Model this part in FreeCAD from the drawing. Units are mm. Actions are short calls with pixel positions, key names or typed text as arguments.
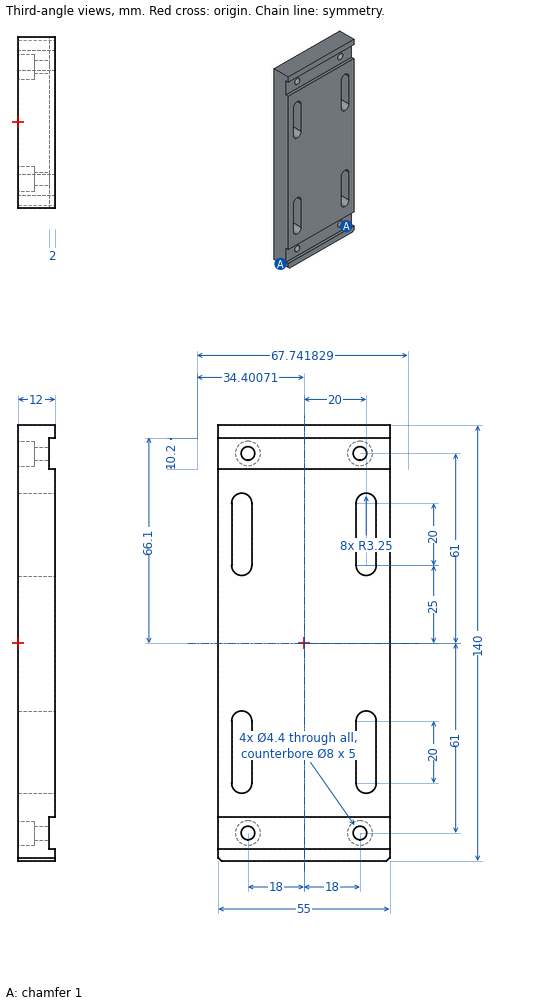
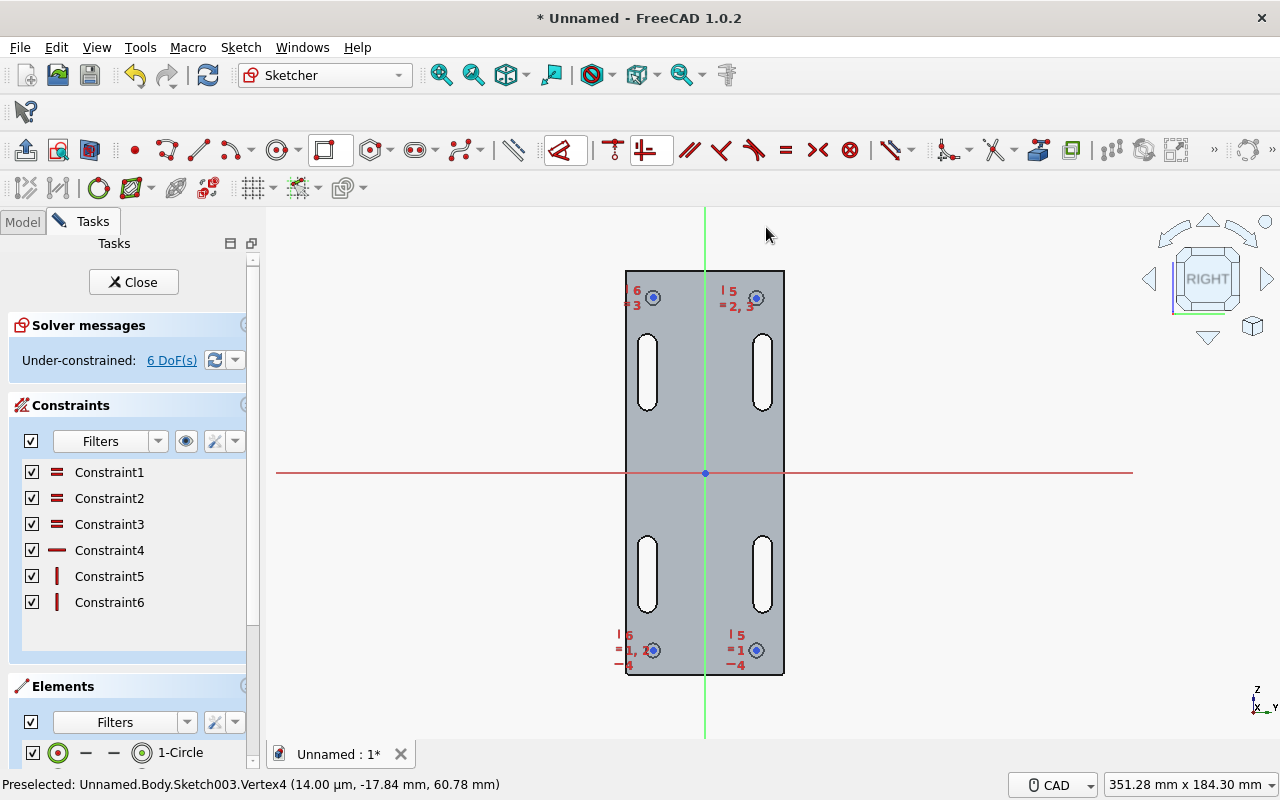
click(757, 298)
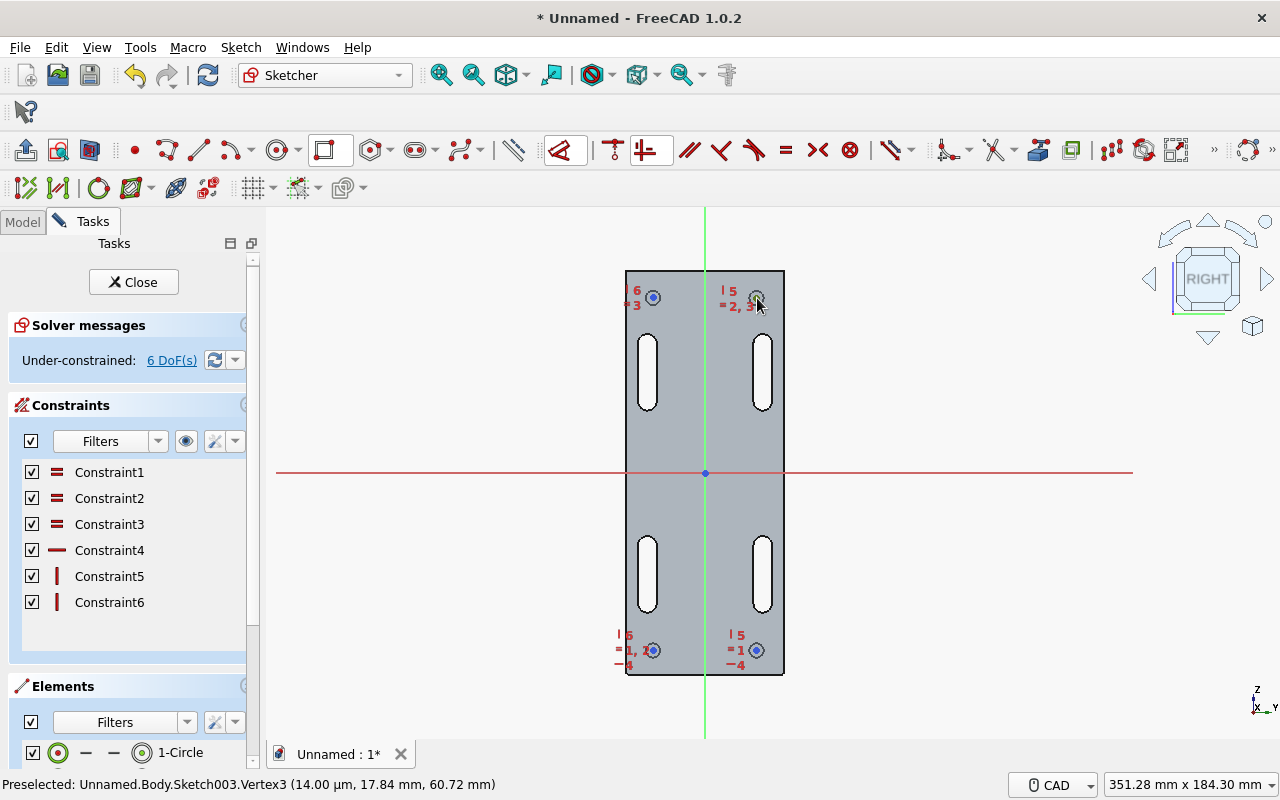
click(653, 298)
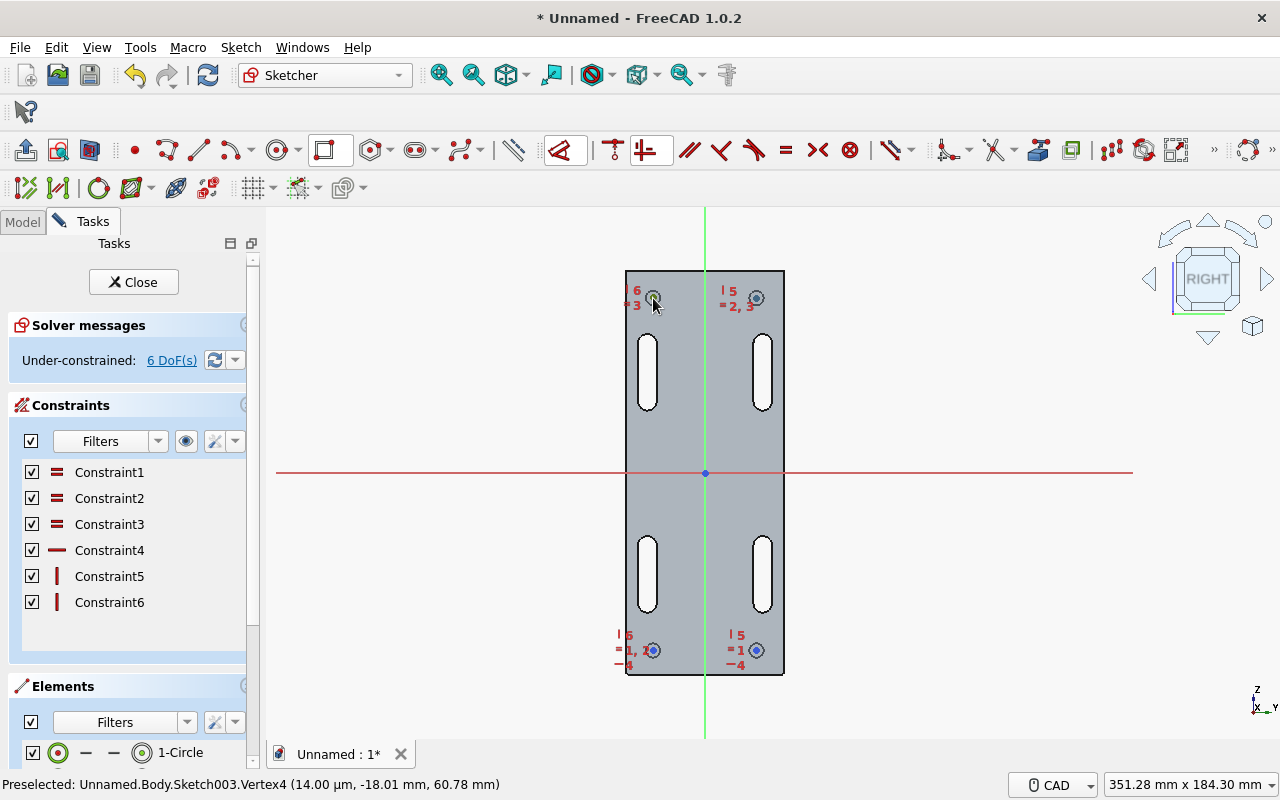
click(668, 150)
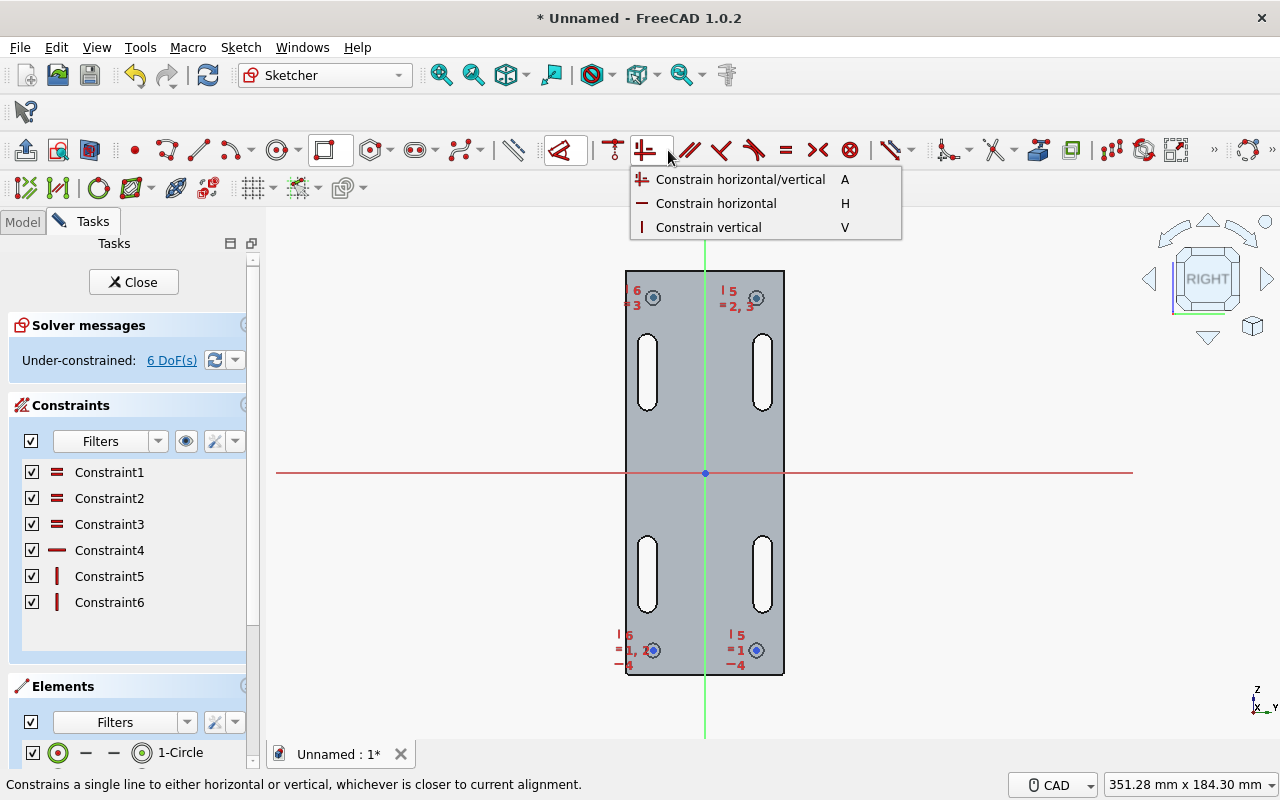
click(766, 203)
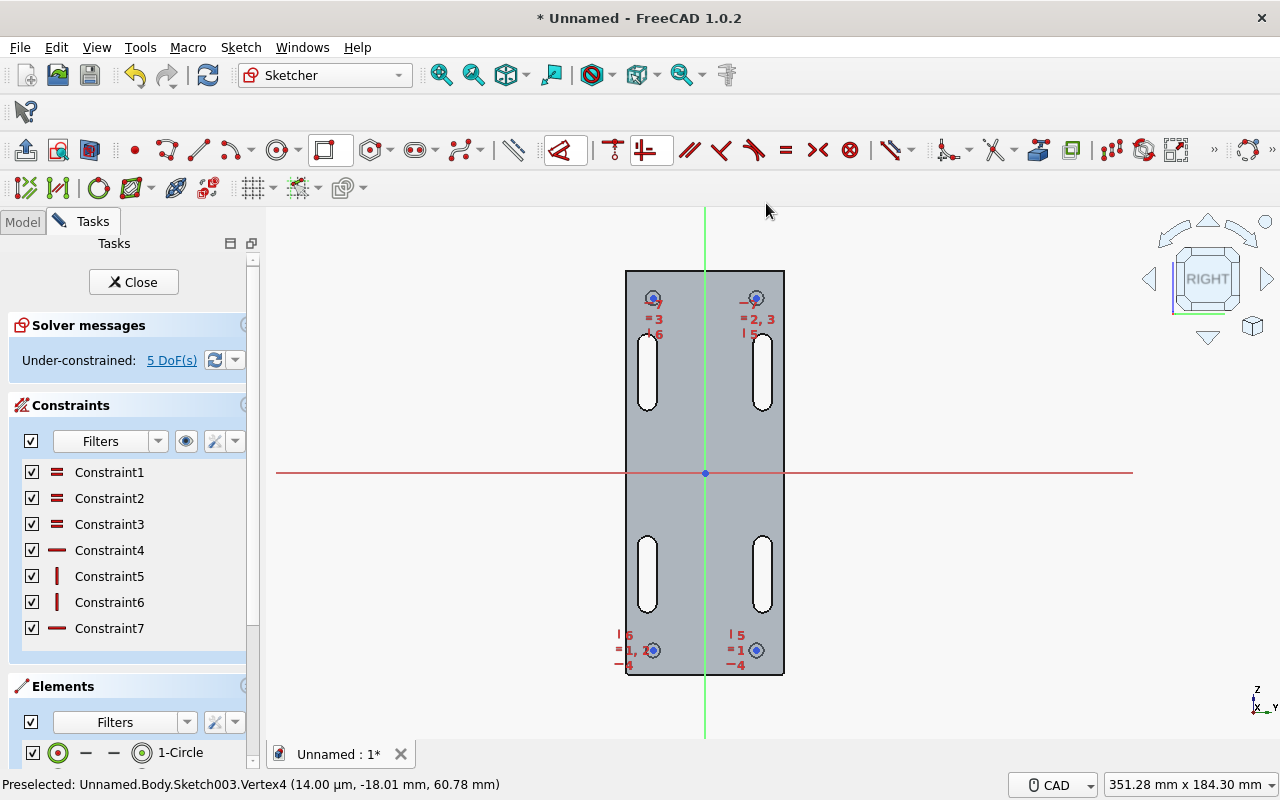
scroll(751, 645, up, 6)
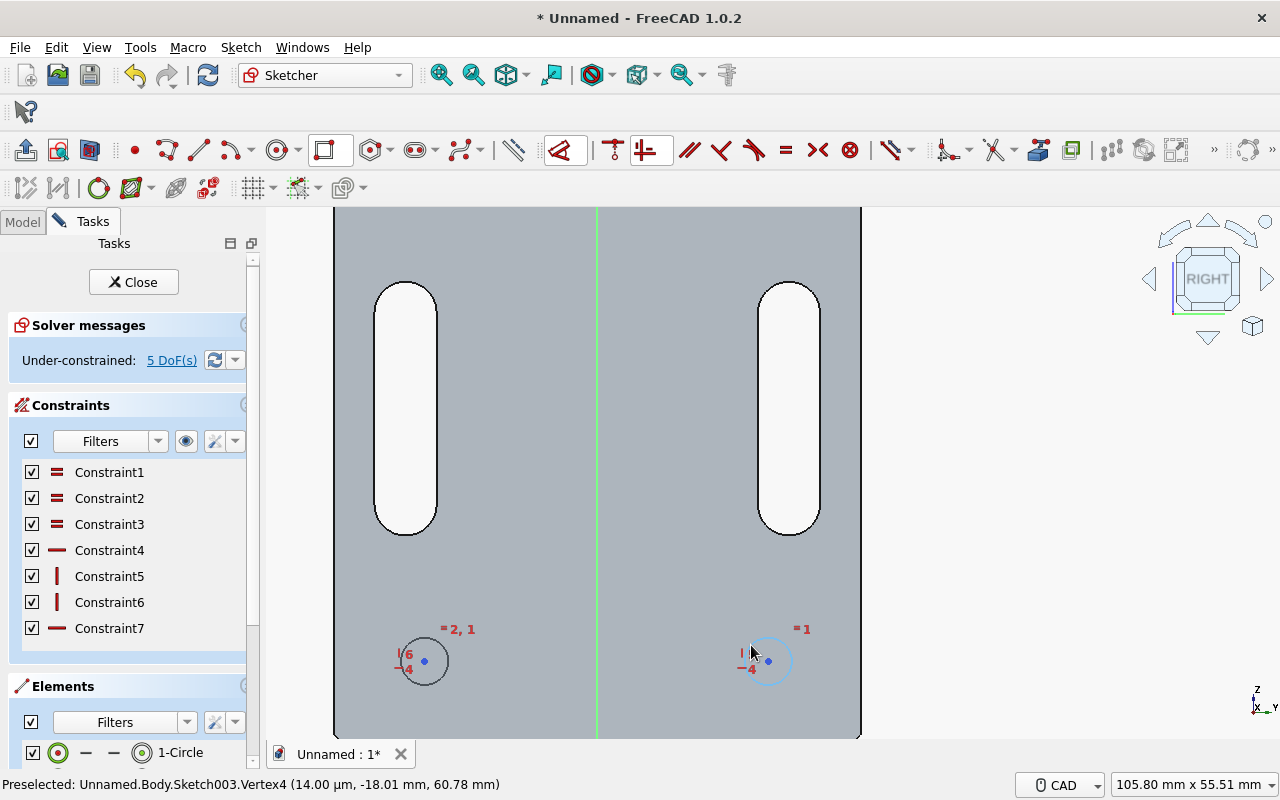
click(752, 645)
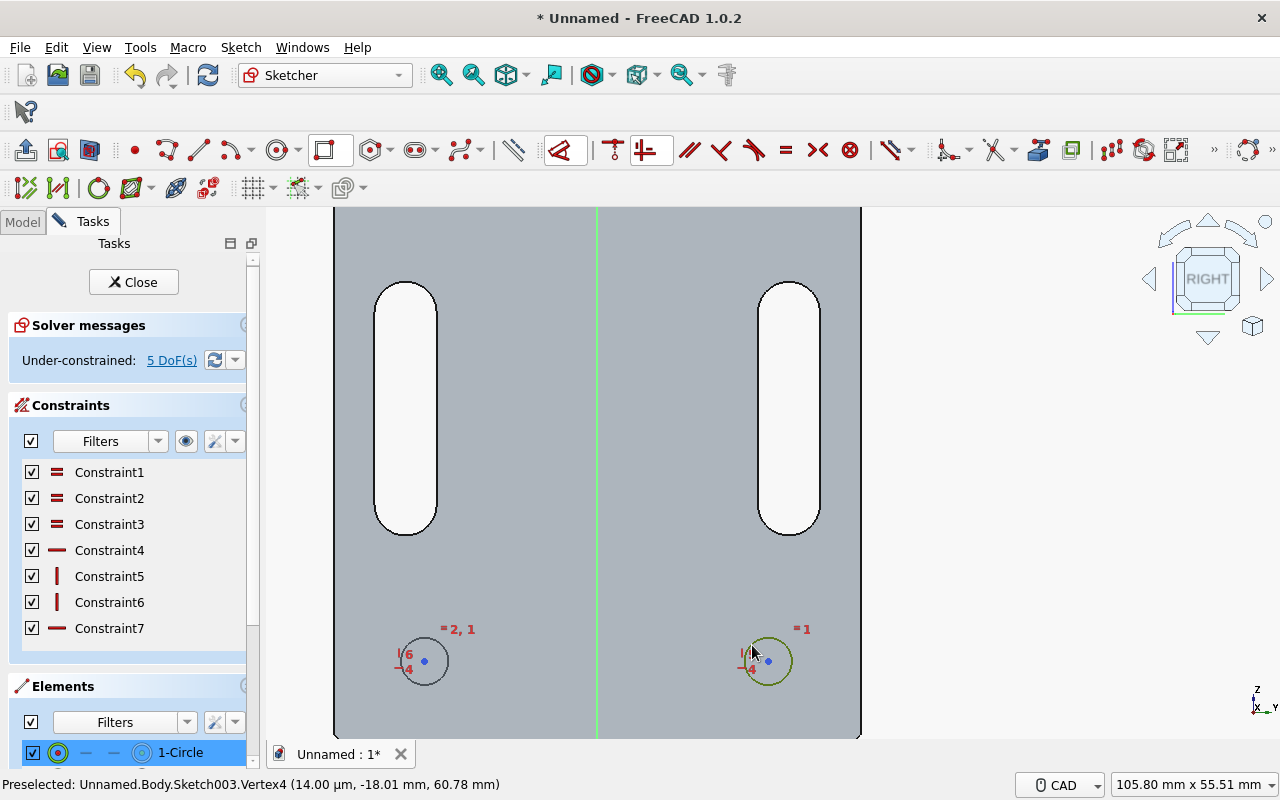
click(582, 150)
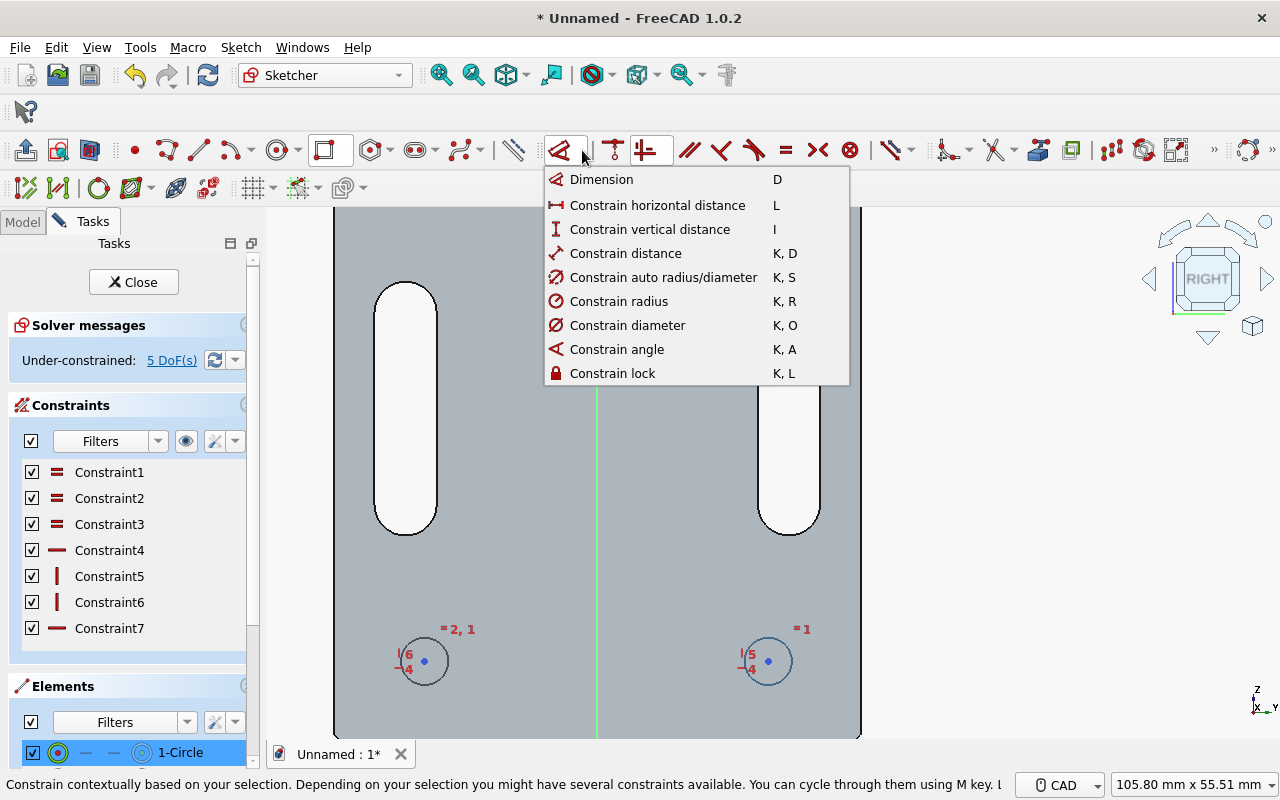
click(697, 325)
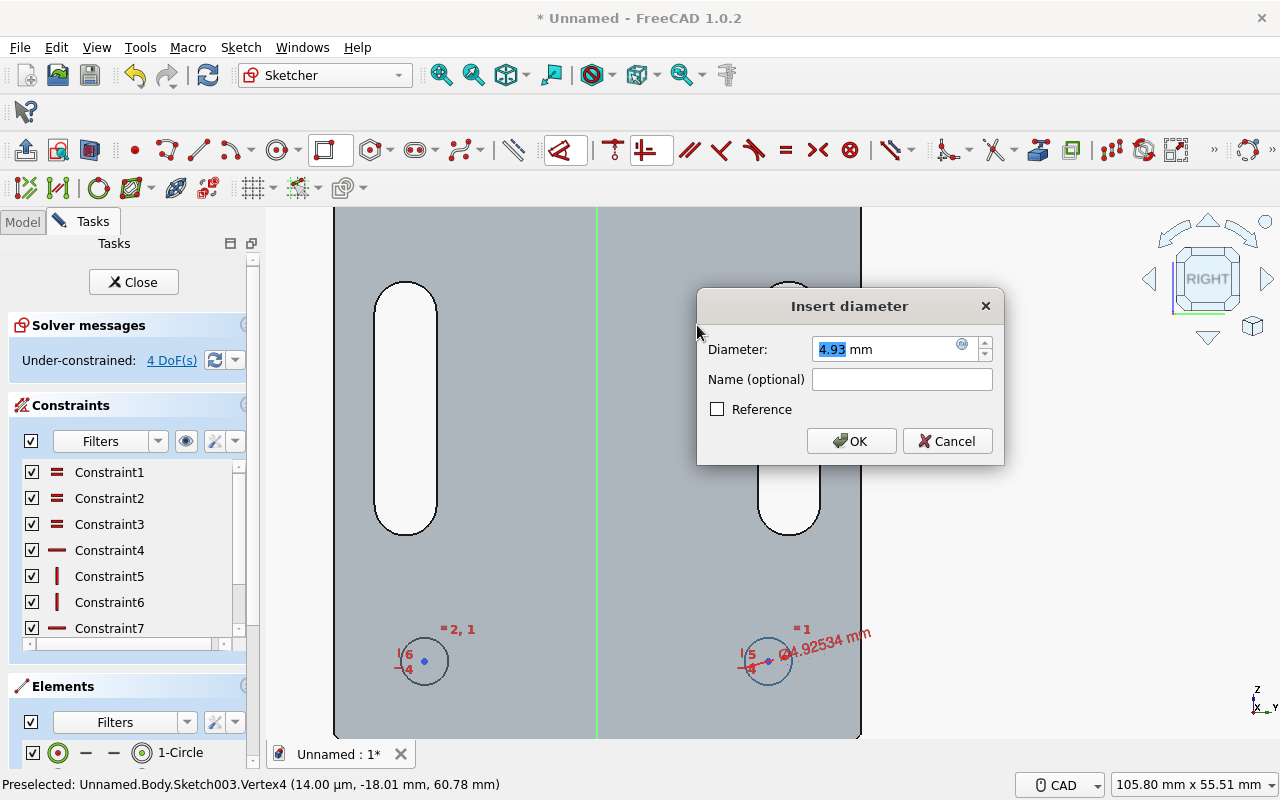
text(4.4)
key(Return)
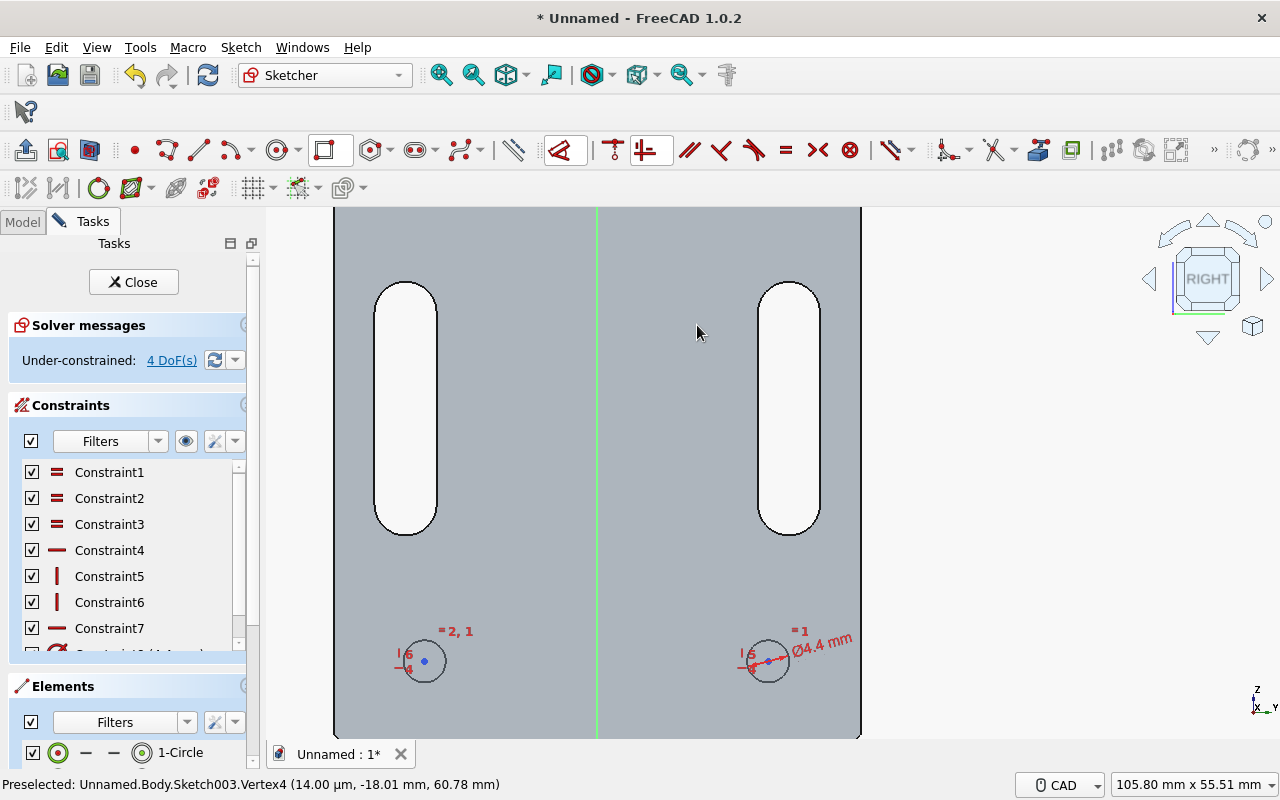
click(768, 661)